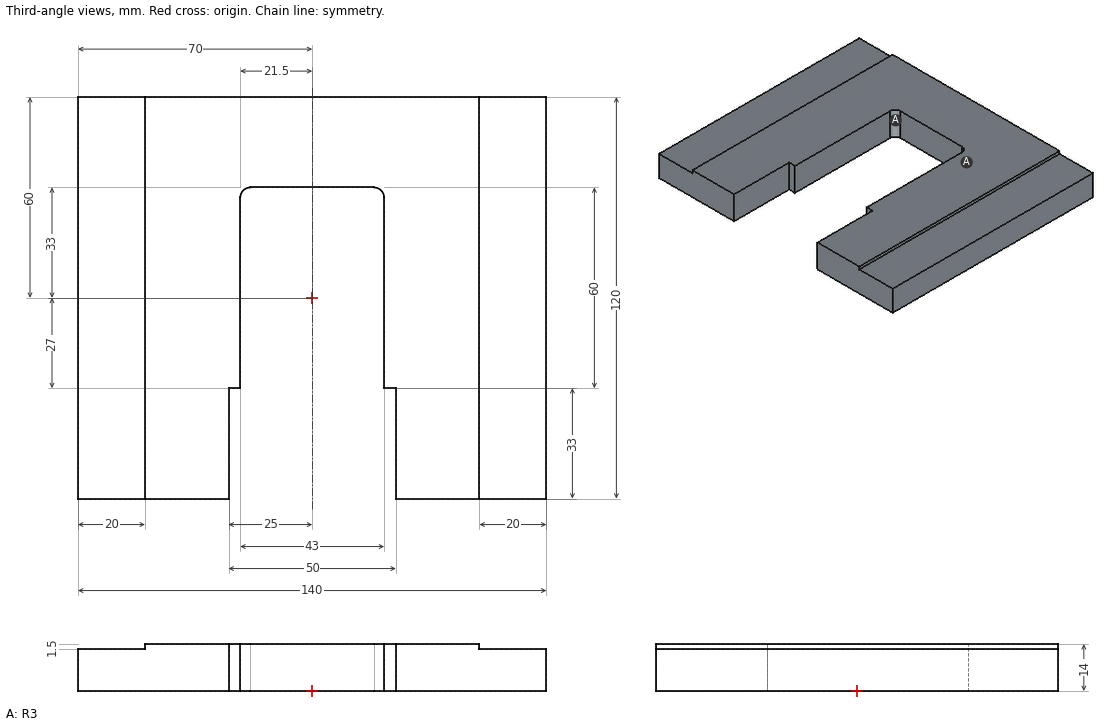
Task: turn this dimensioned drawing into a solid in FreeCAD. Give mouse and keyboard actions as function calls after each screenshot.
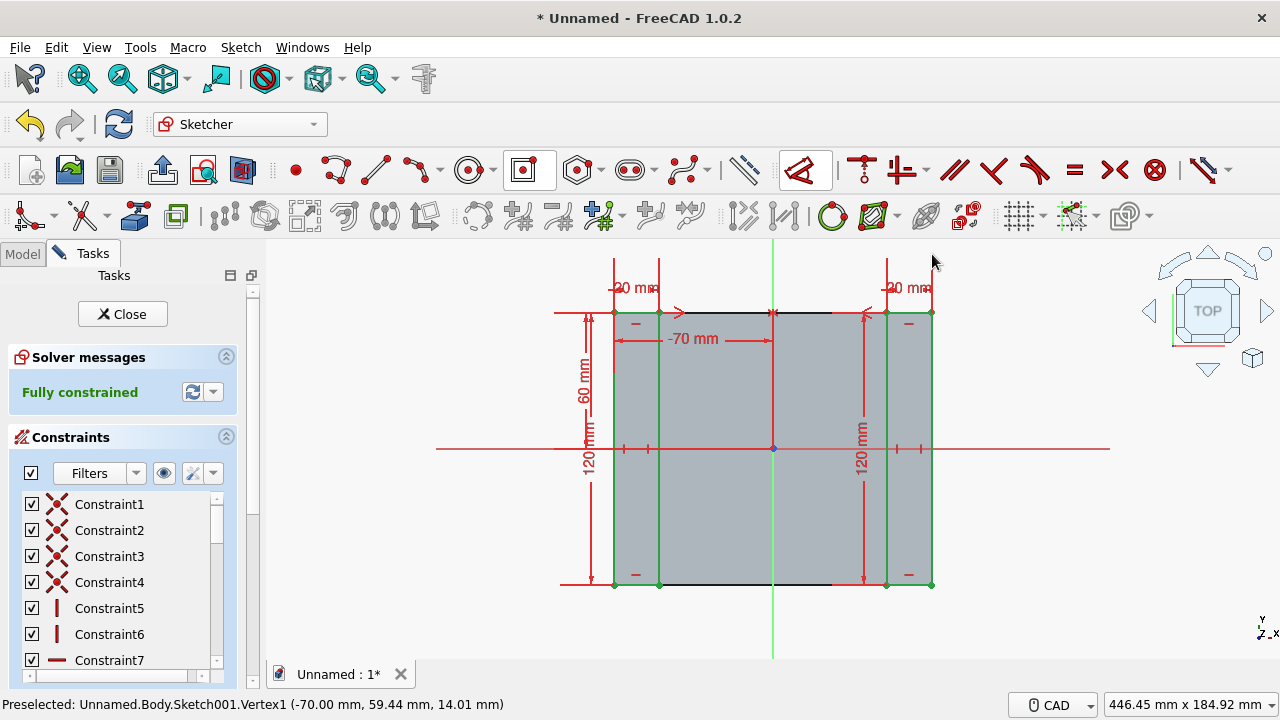
click(123, 314)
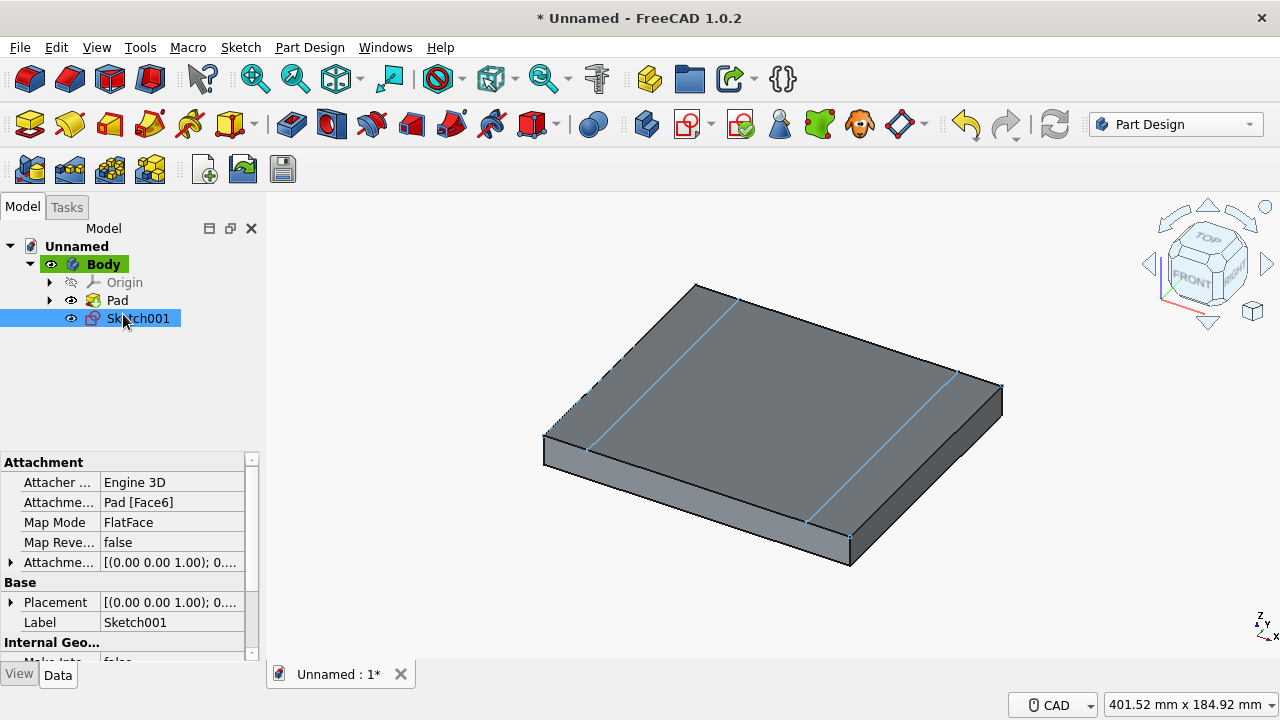
click(292, 124)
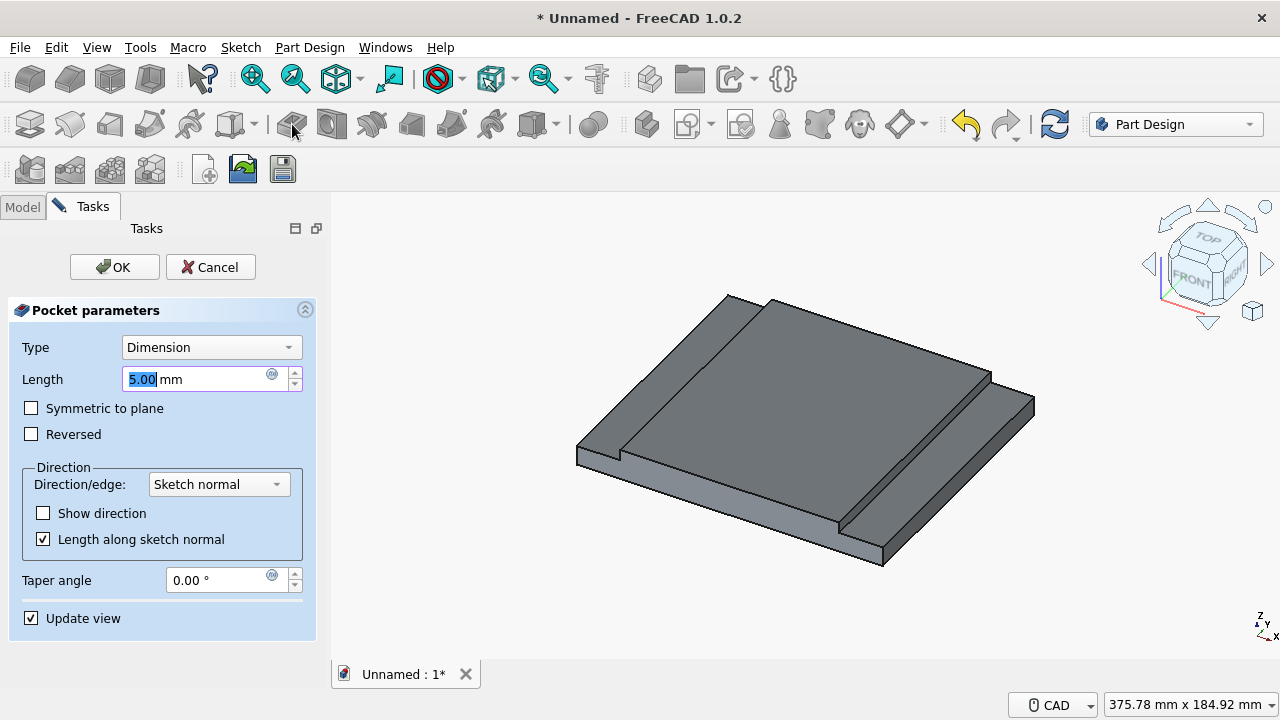
text(1.5)
key(Tab)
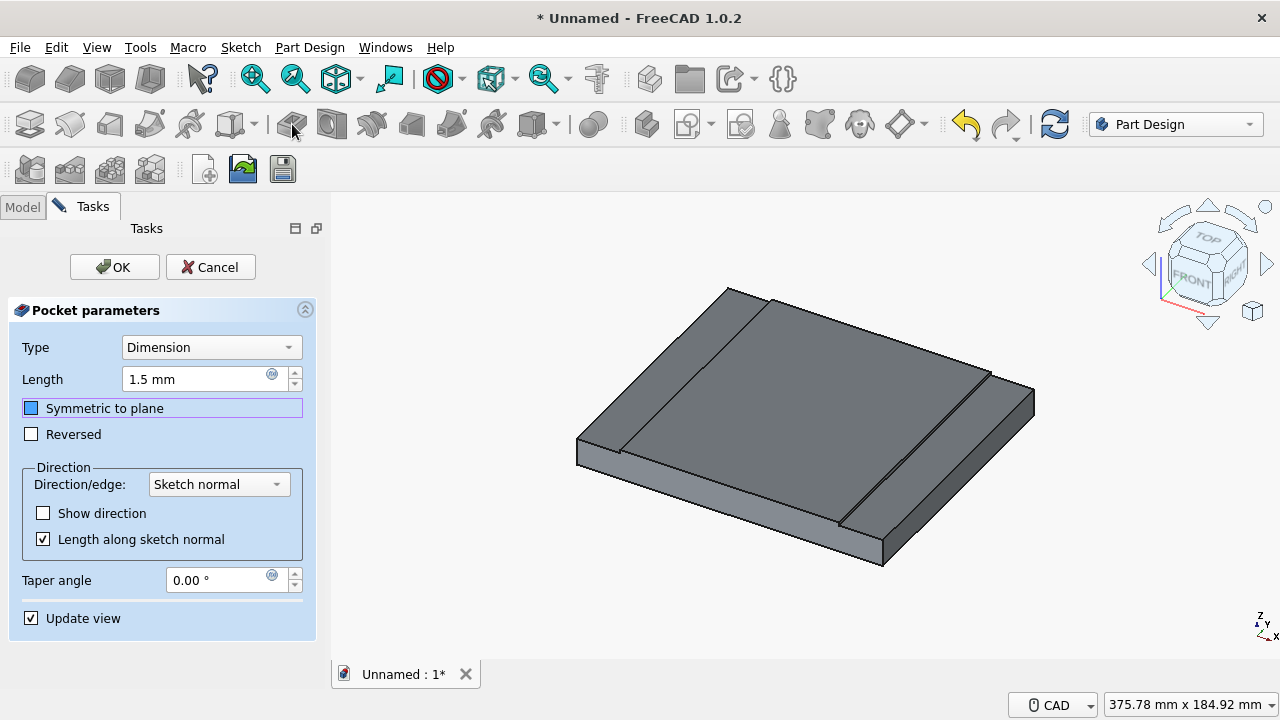
click(115, 267)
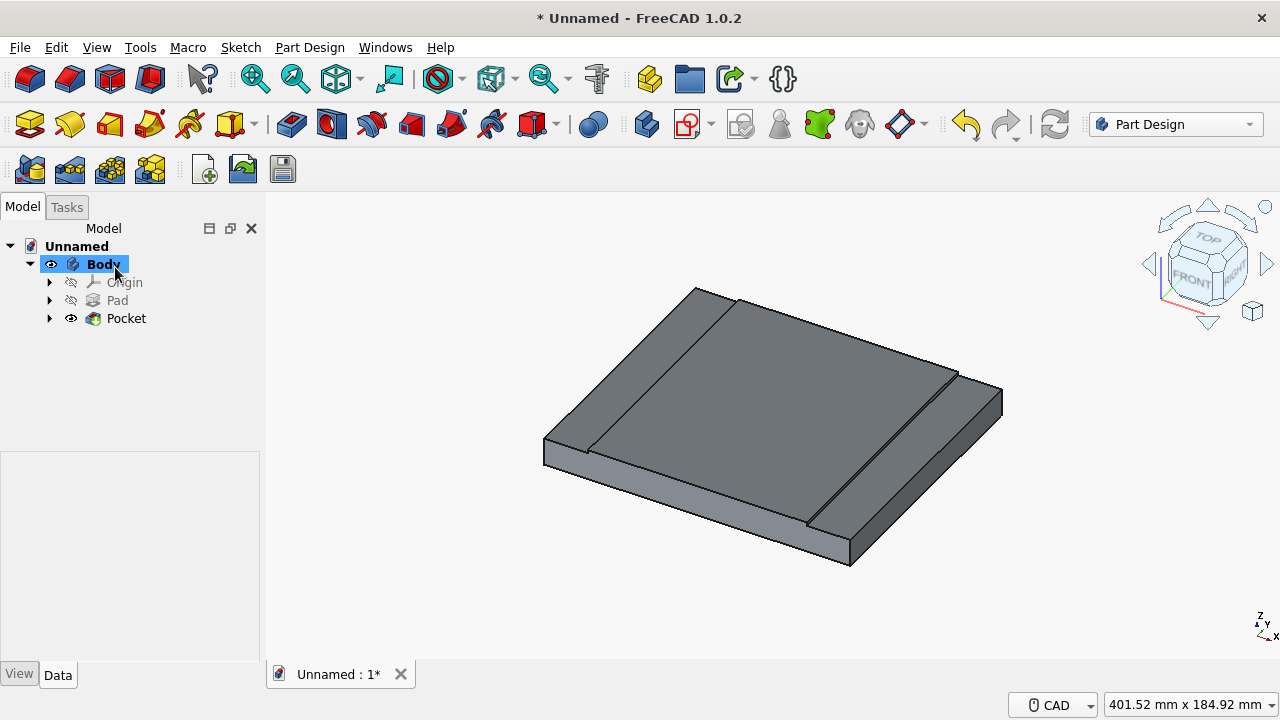
click(773, 410)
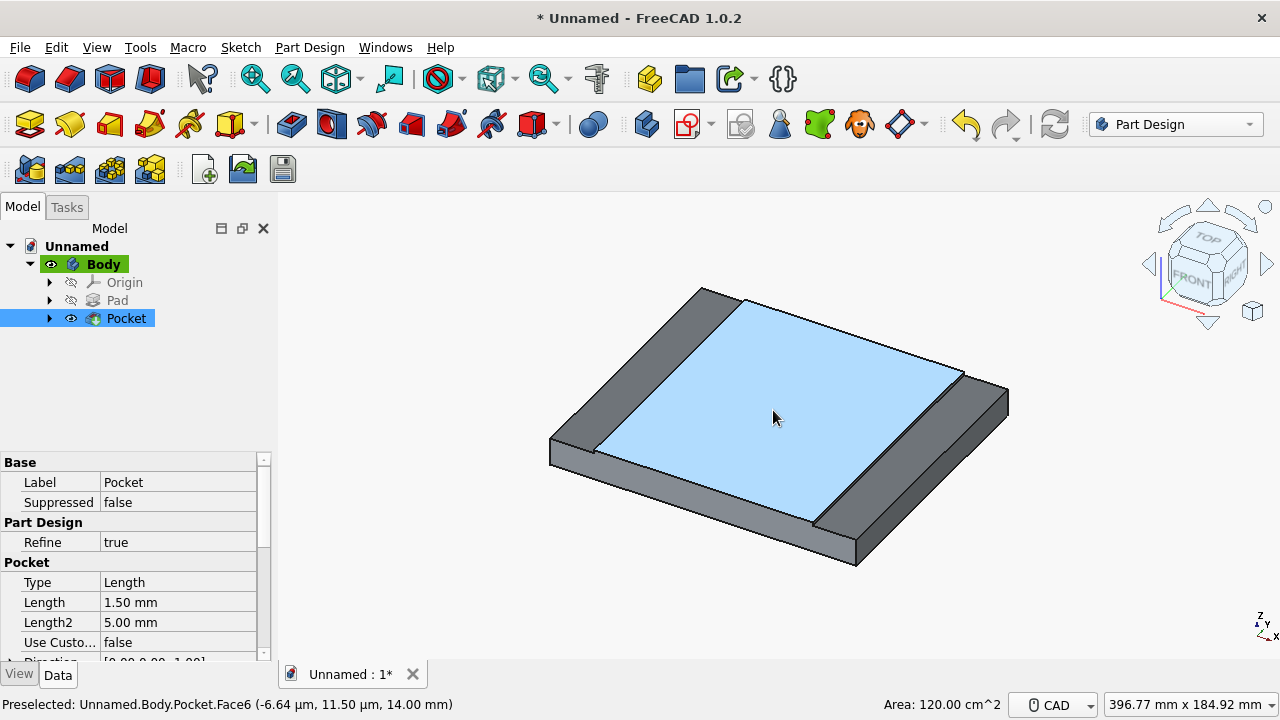
click(688, 124)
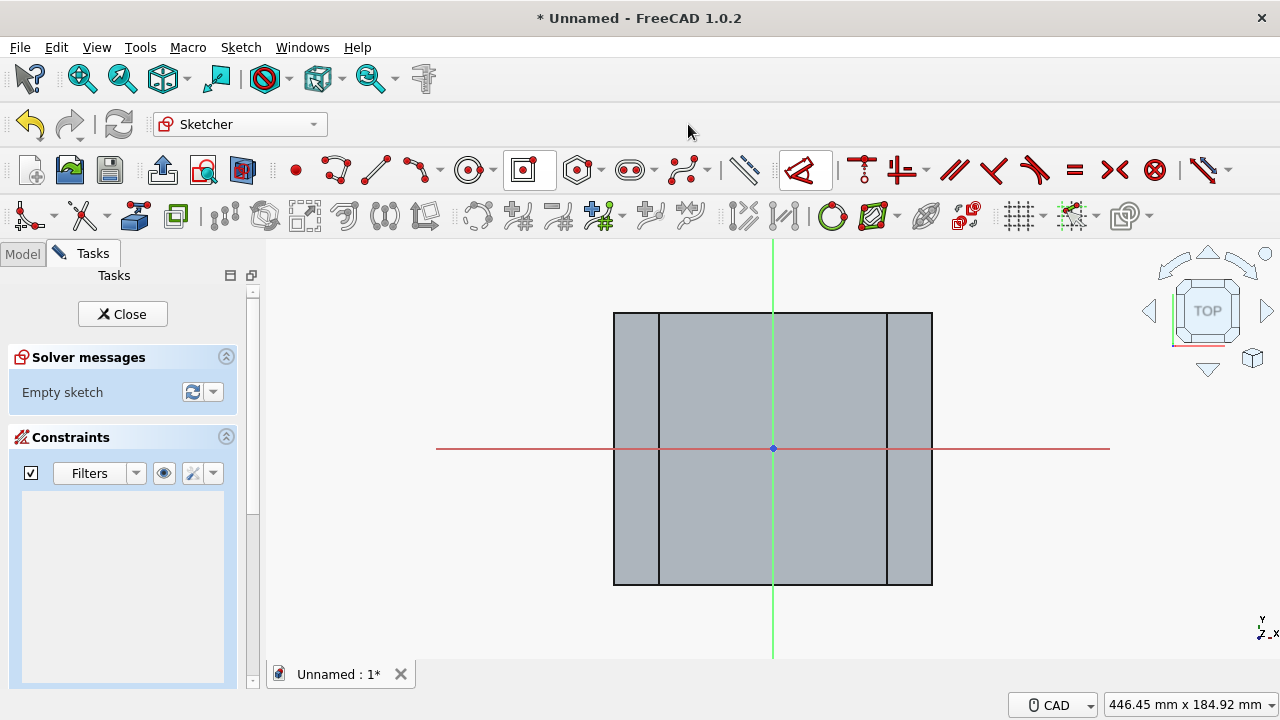
scroll(856, 600, up, 3)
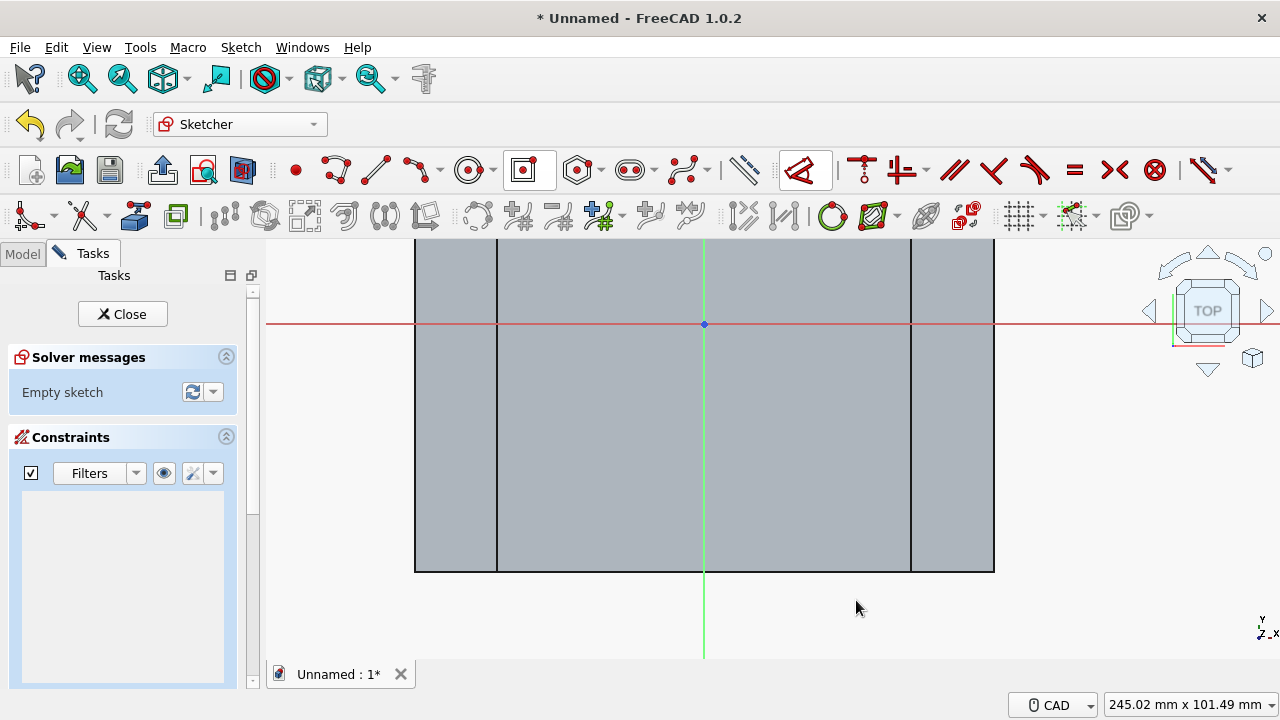
key(g)
key(r)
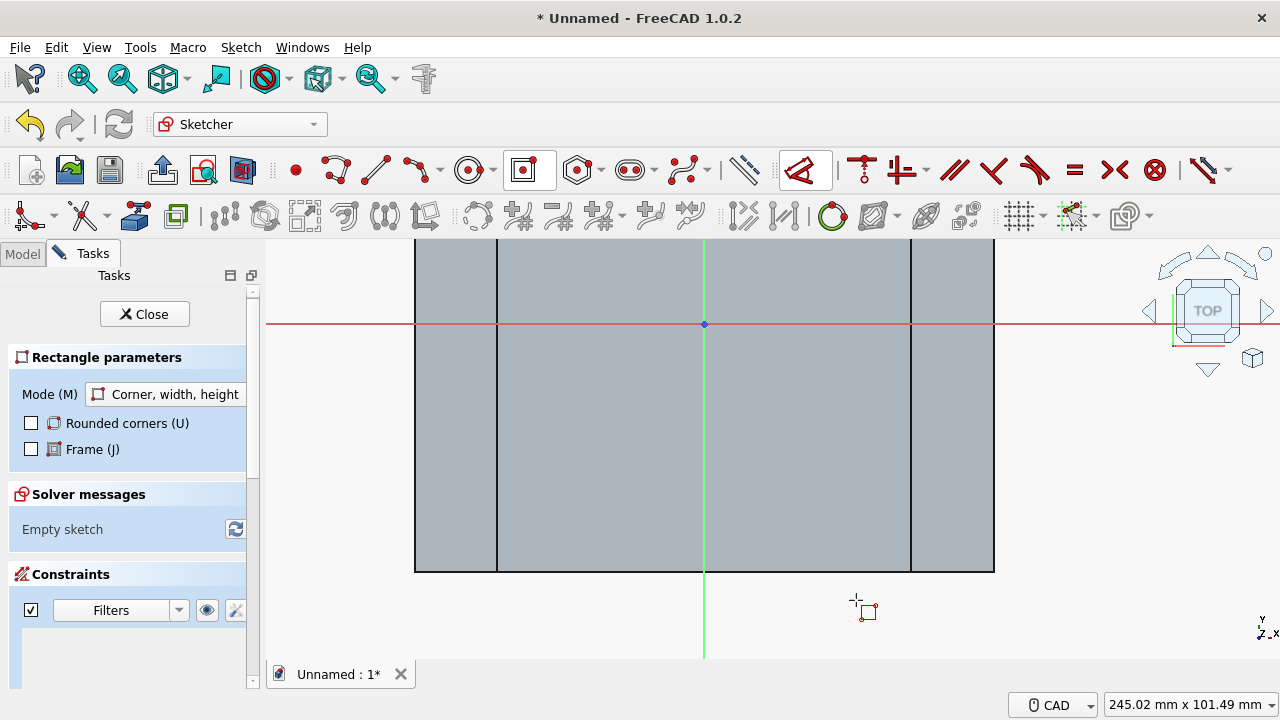
click(601, 436)
move(808, 572)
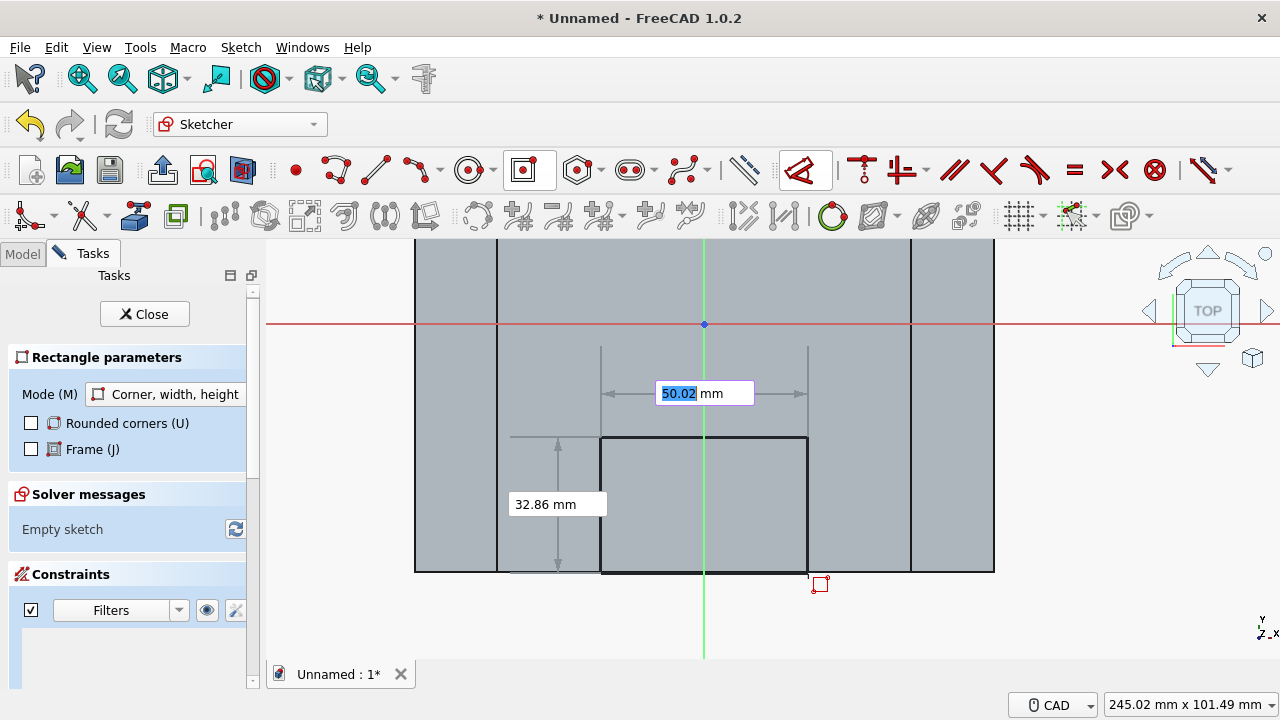
text(50)
key(Tab)
text(33)
key(Return)
key(Escape)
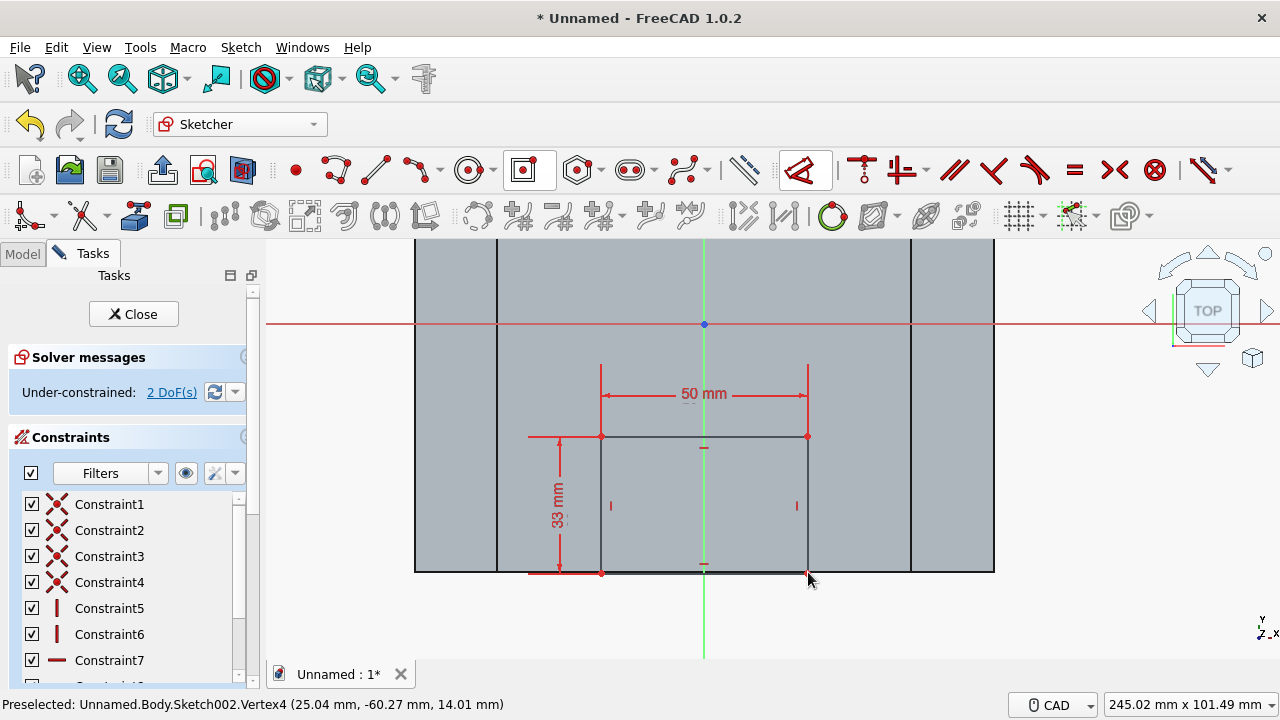
click(601, 437)